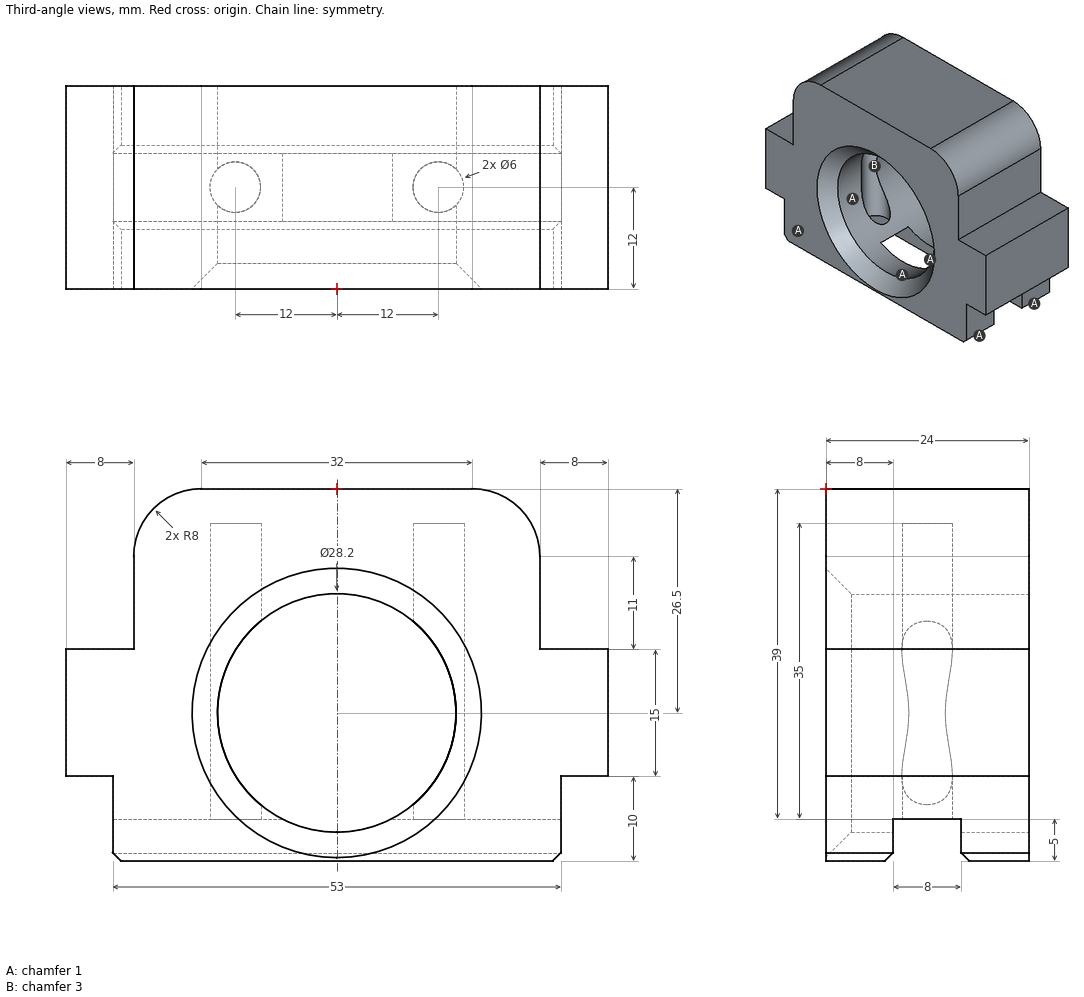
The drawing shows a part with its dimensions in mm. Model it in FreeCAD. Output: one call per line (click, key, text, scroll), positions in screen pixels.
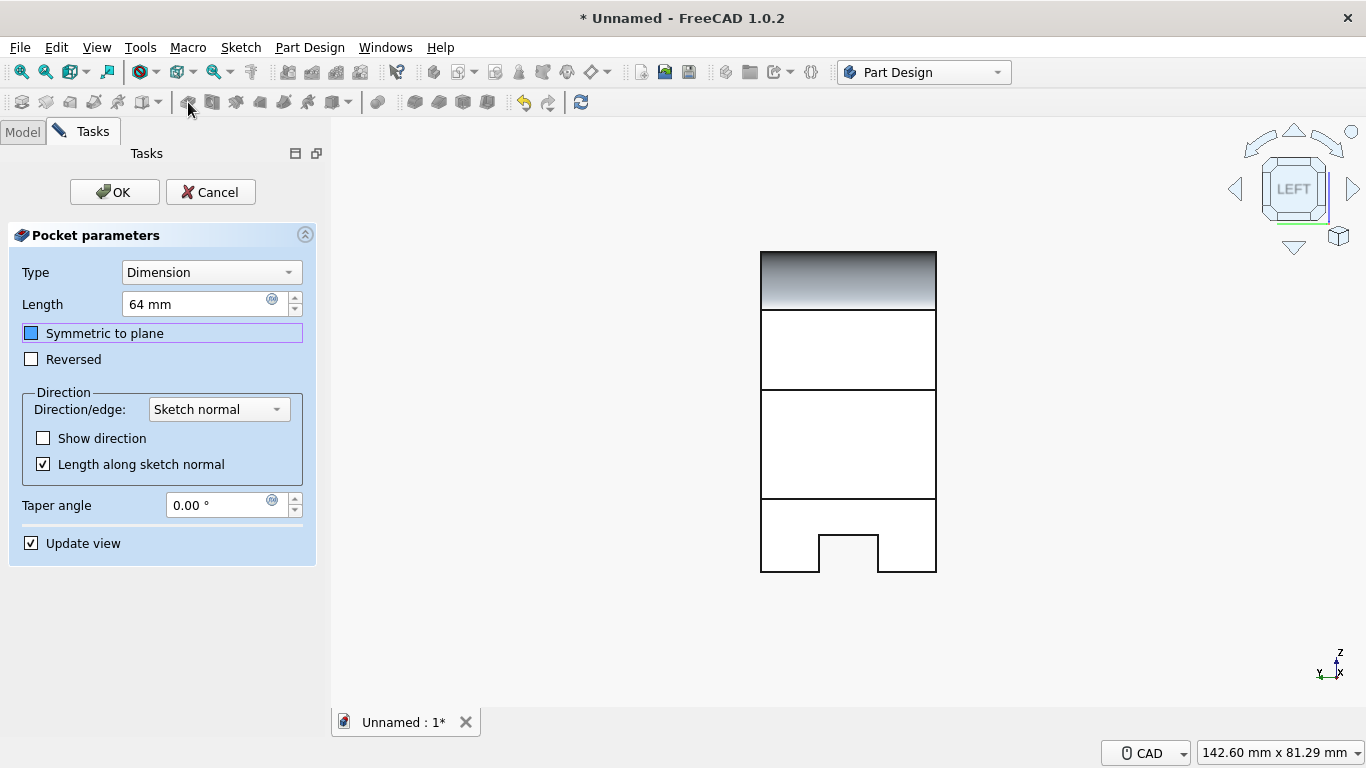
click(115, 192)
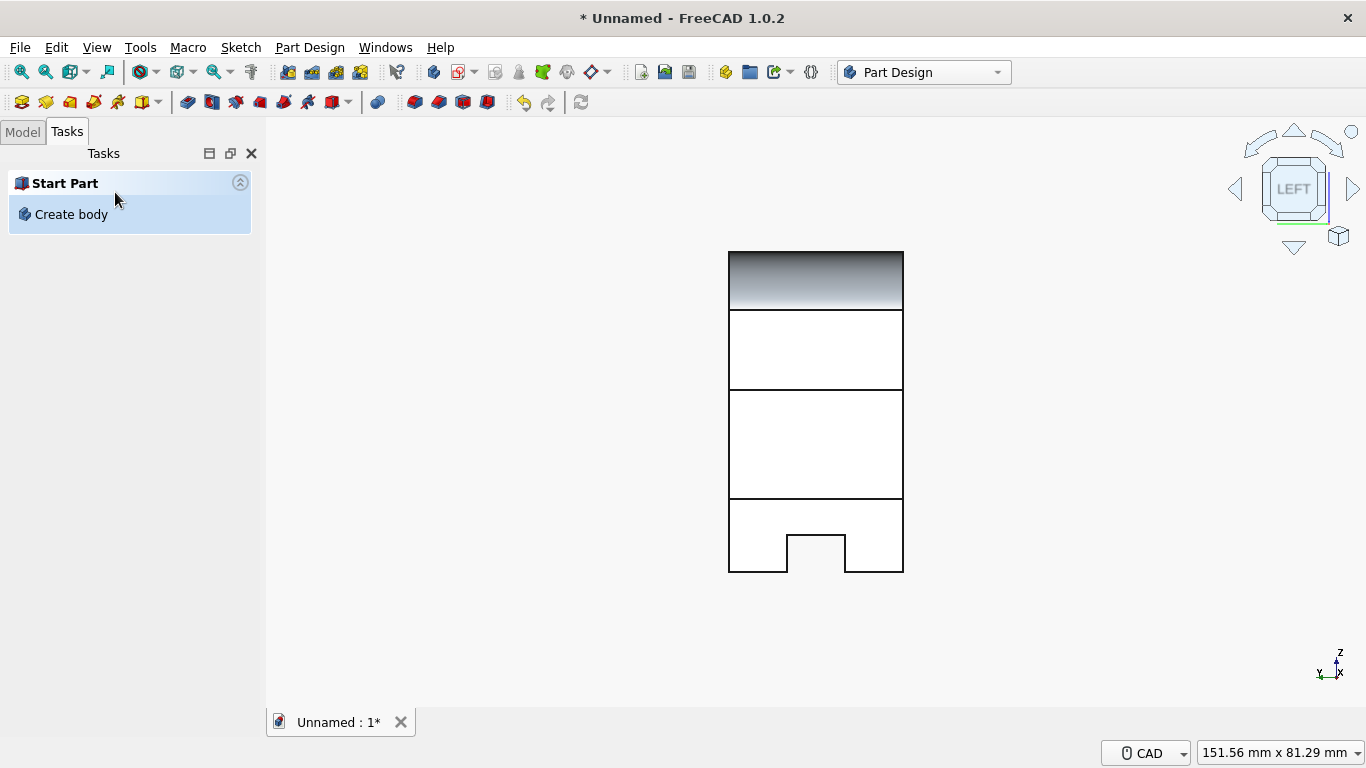
key(5)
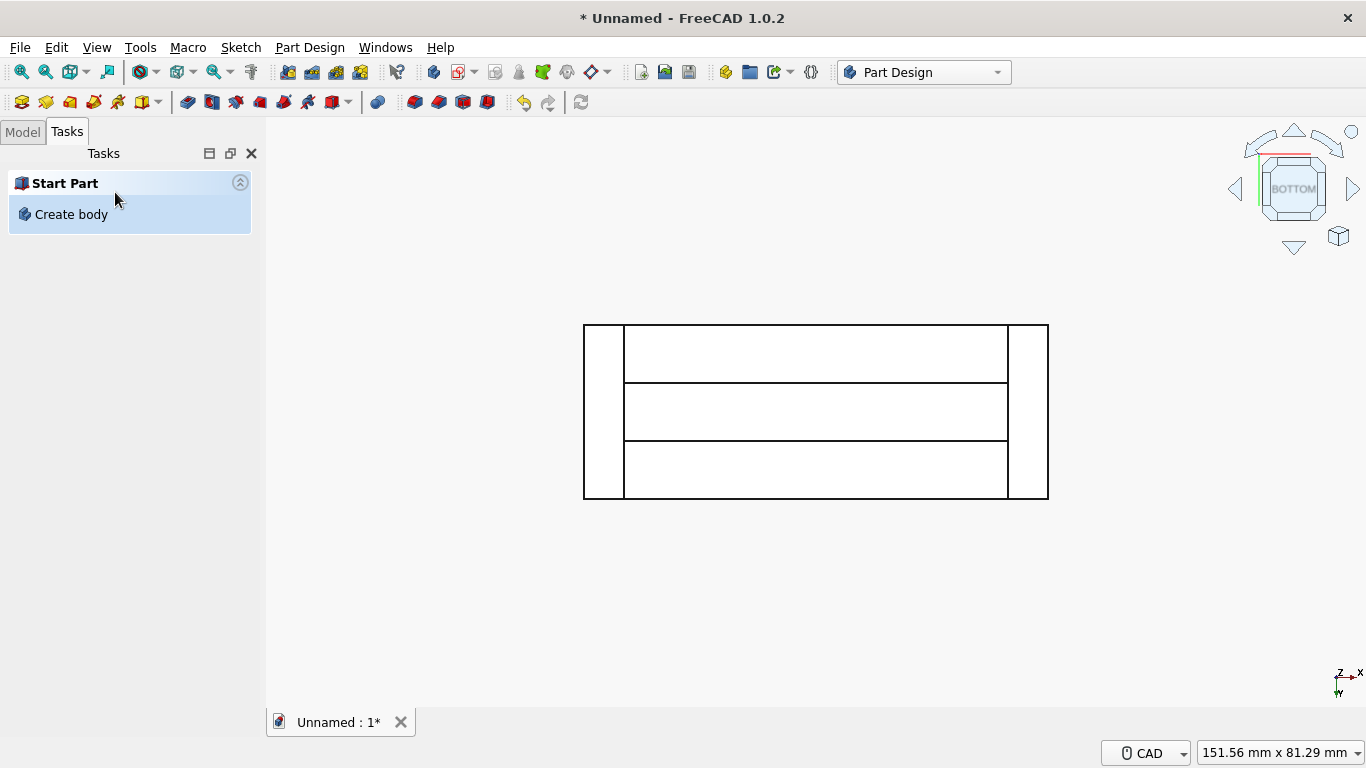
click(22, 72)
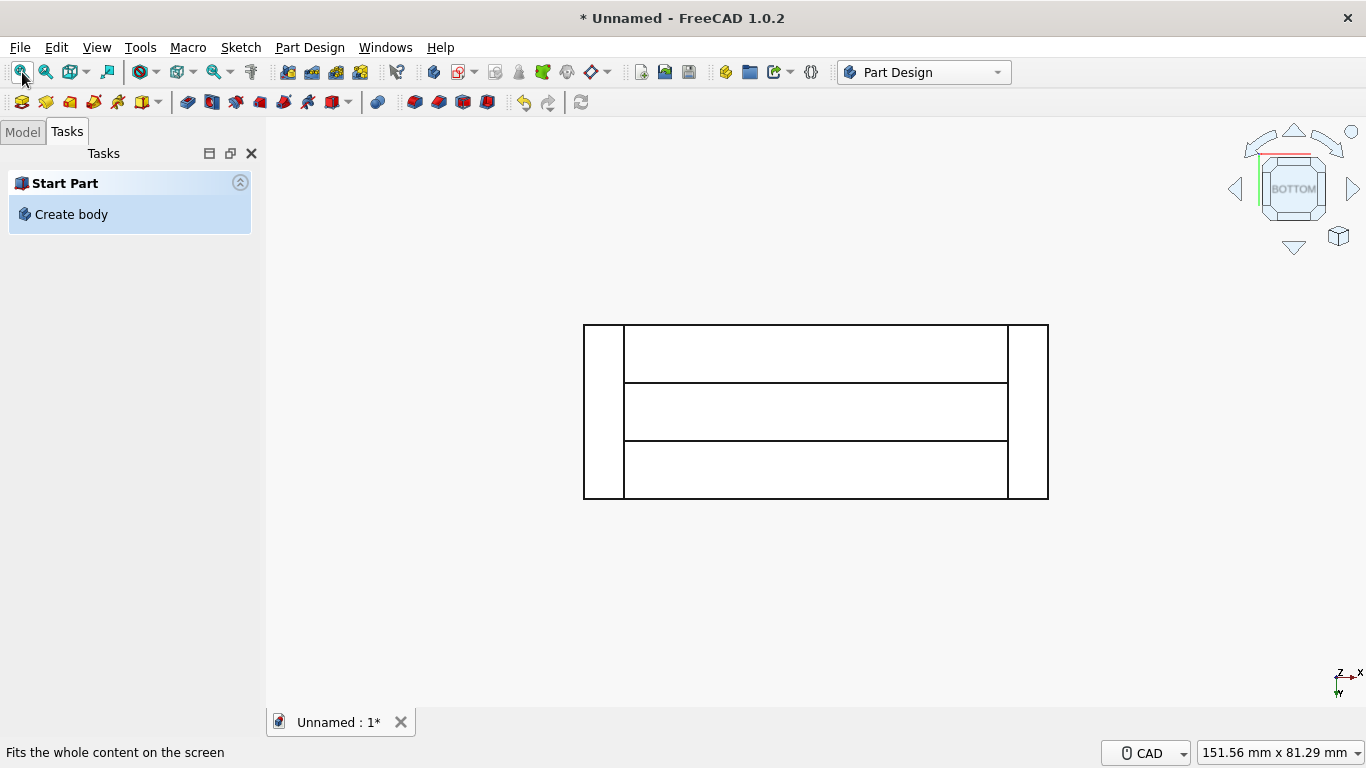
click(926, 411)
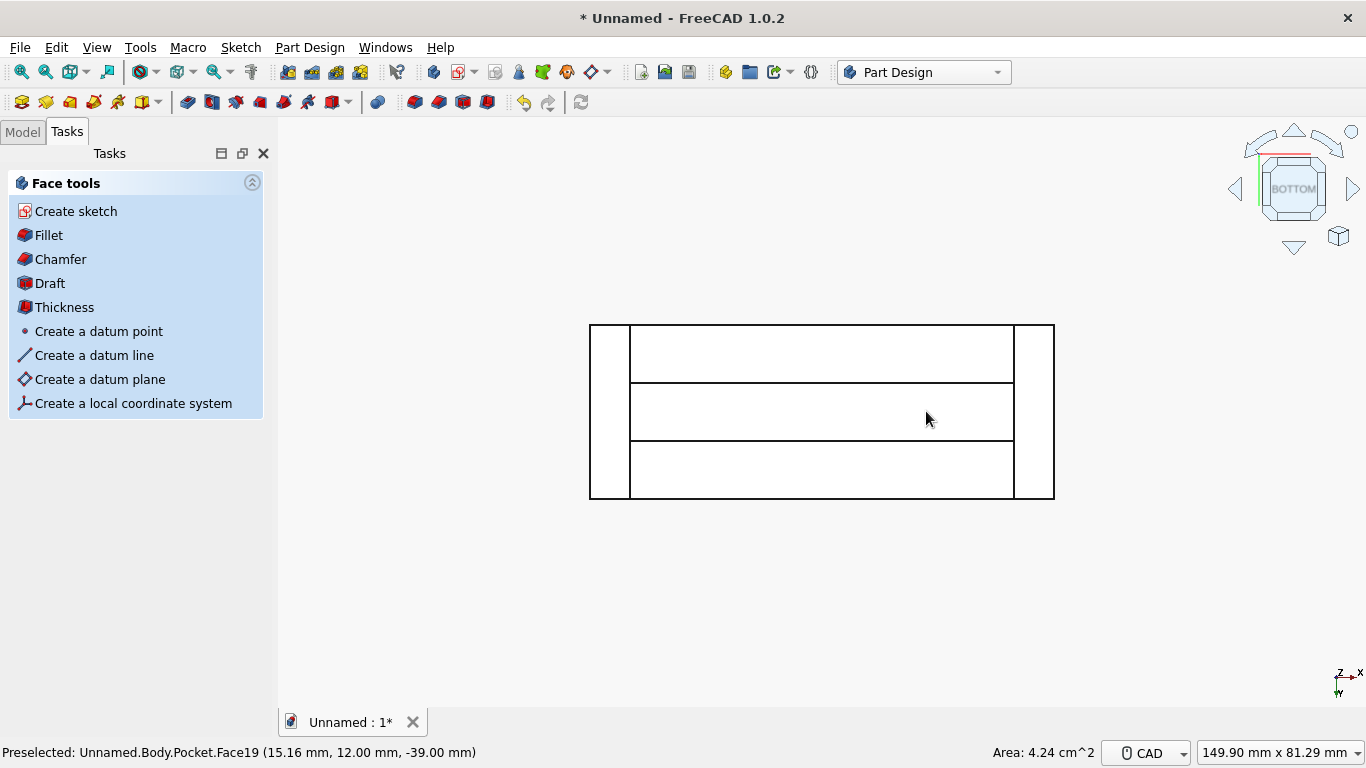
click(458, 72)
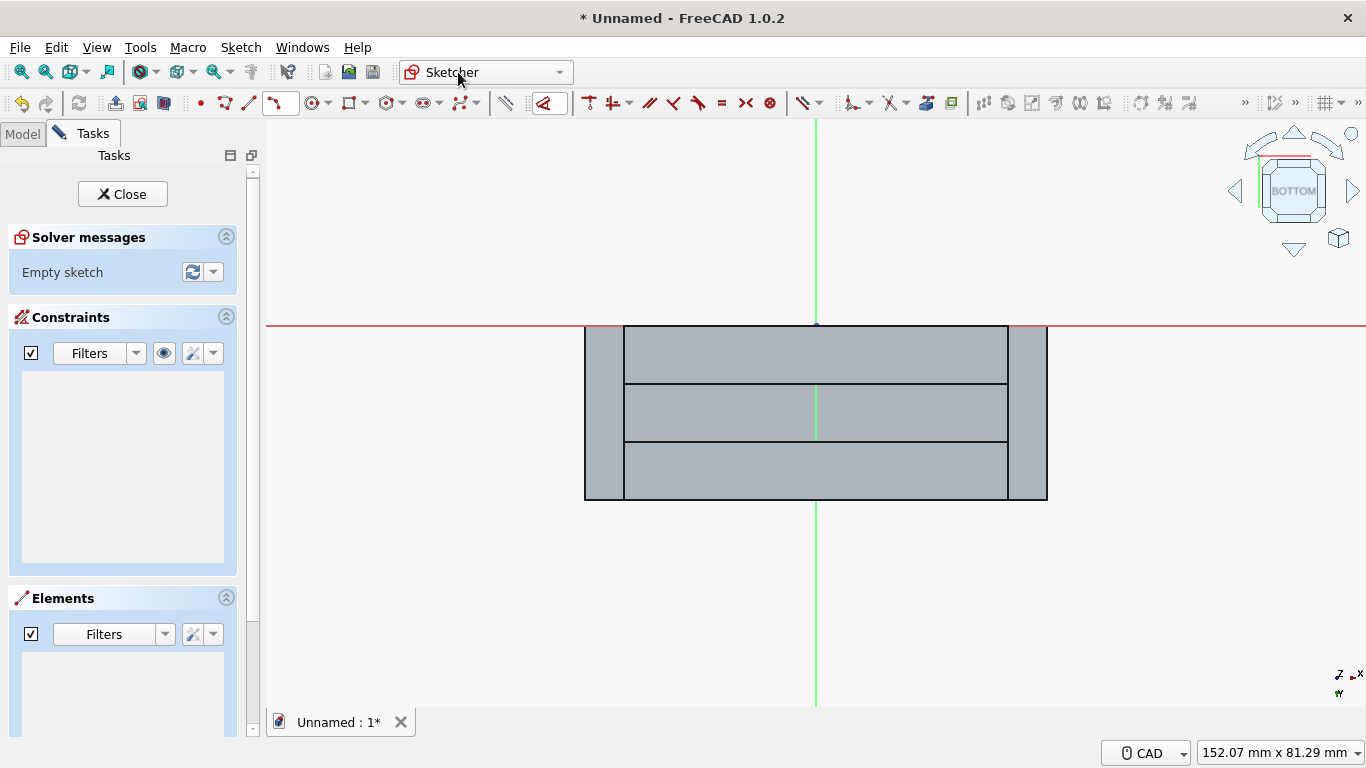
scroll(856, 362, up, 5)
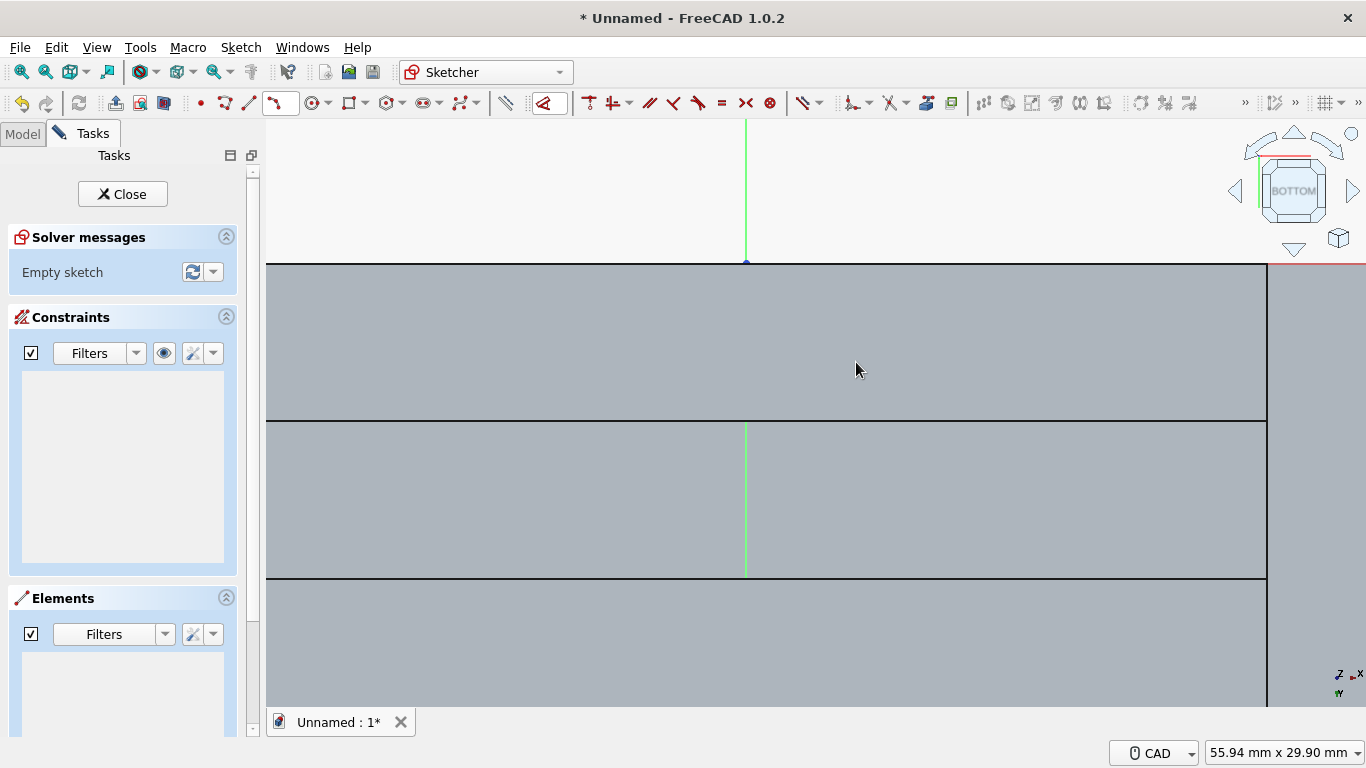
click(312, 104)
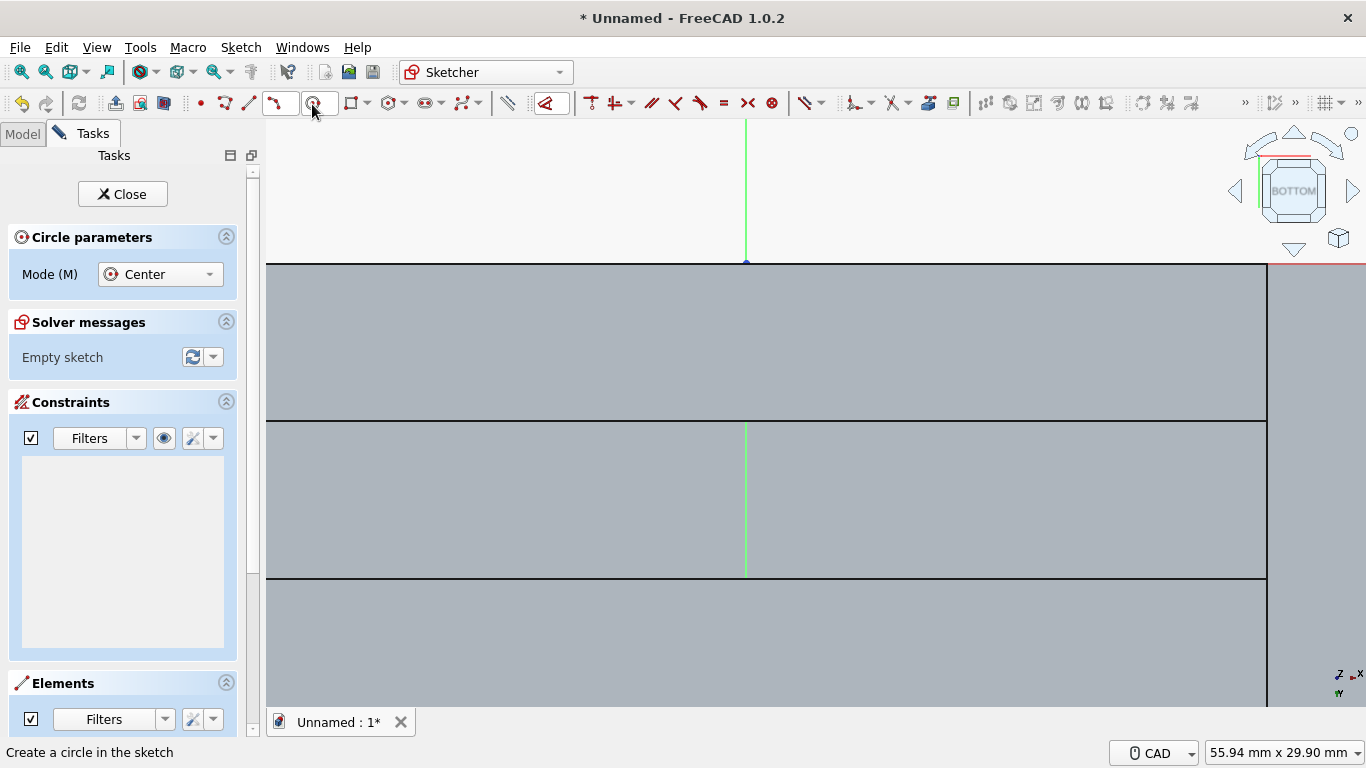
click(982, 500)
move(1024, 458)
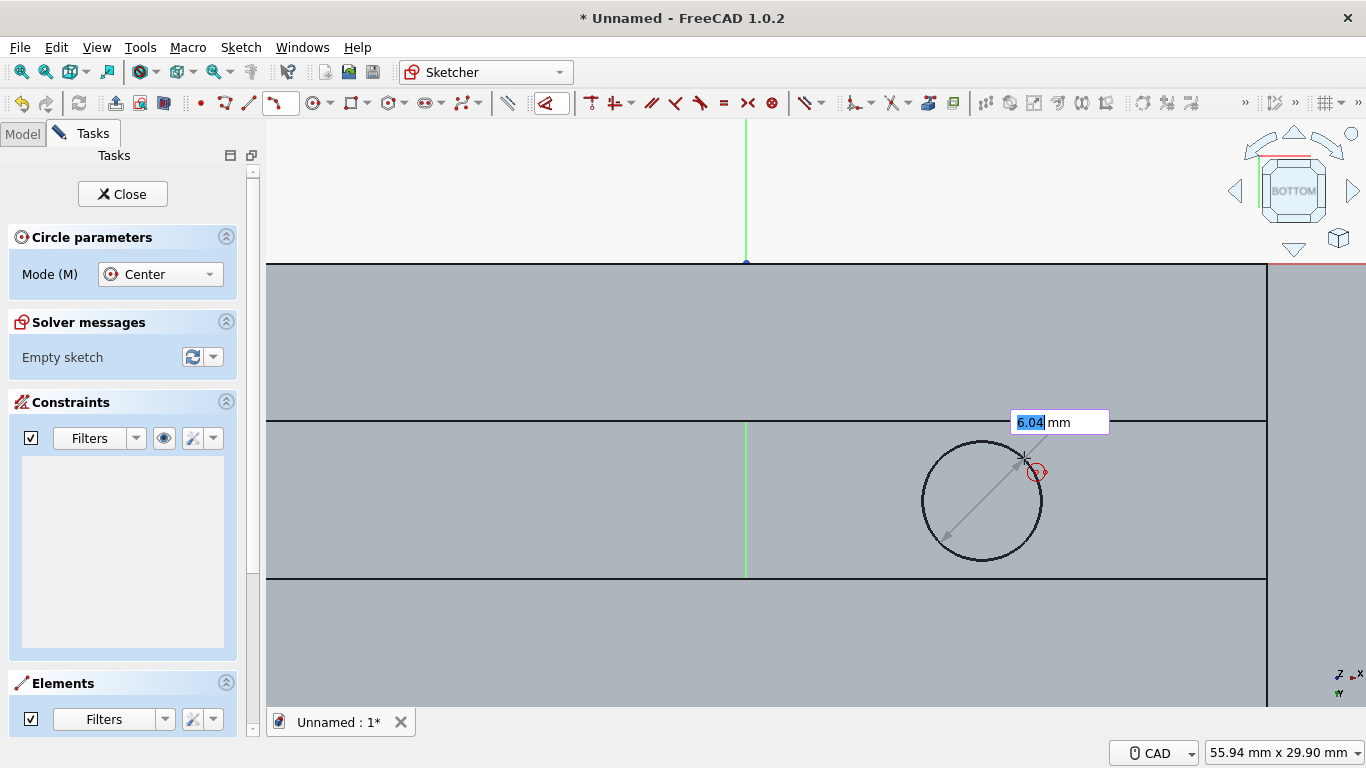
text(6)
key(Return)